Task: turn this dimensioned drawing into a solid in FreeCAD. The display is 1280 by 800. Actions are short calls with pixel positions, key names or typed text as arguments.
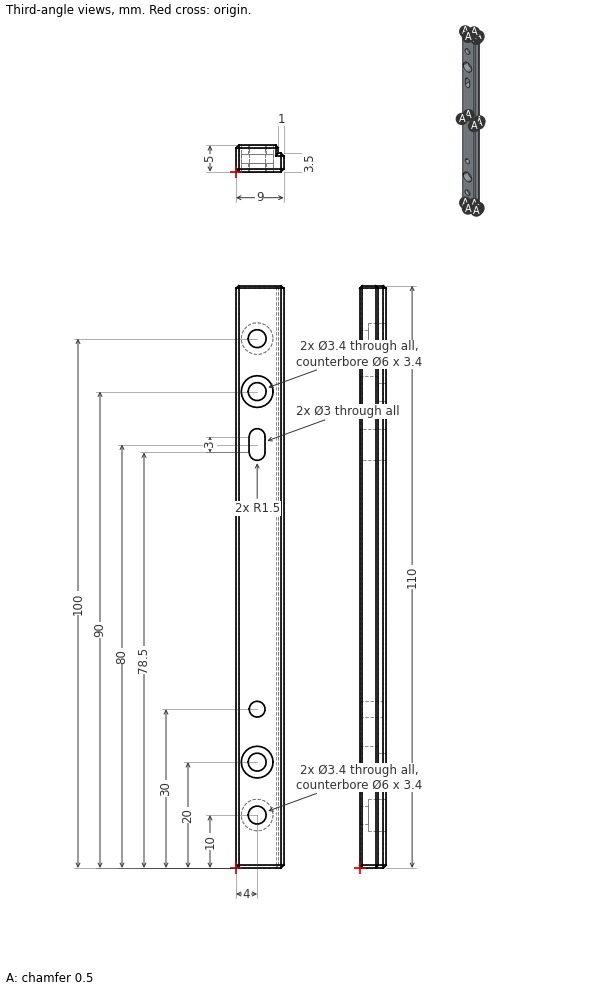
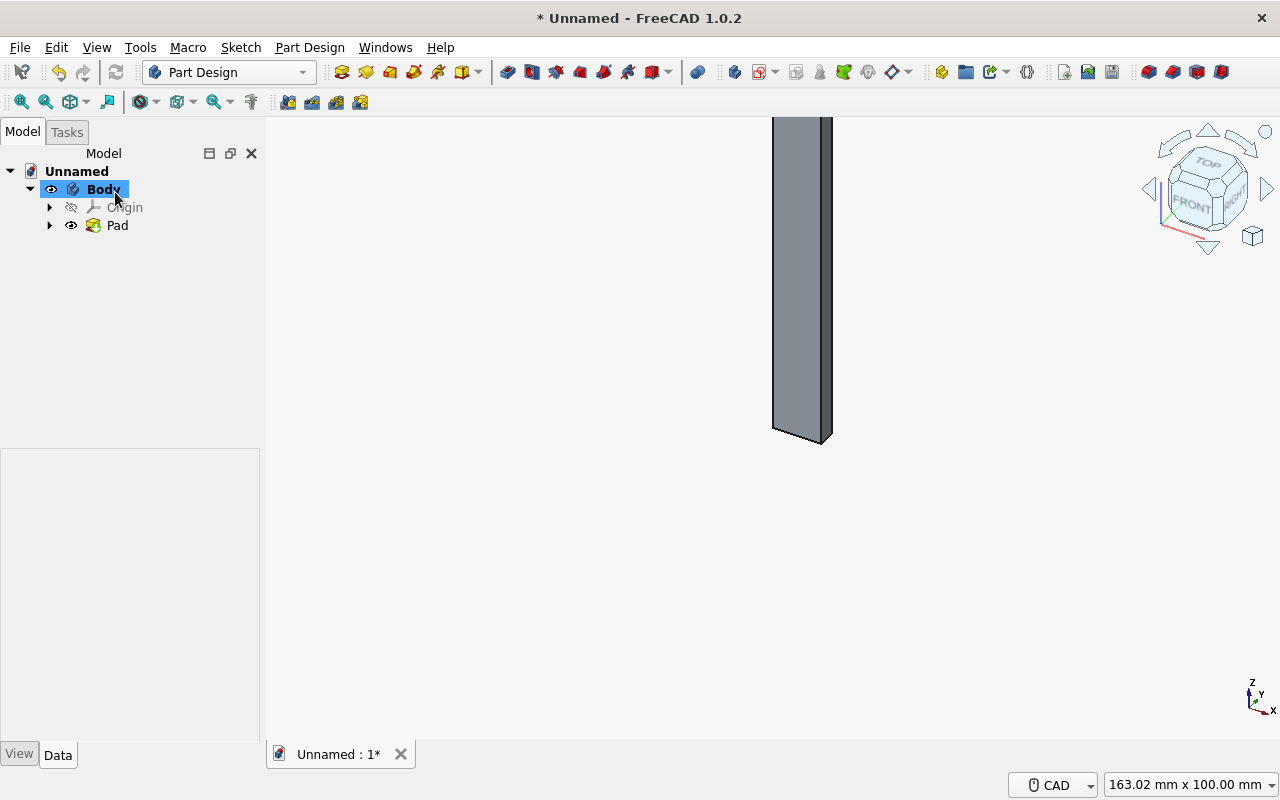
key(v)
key(f)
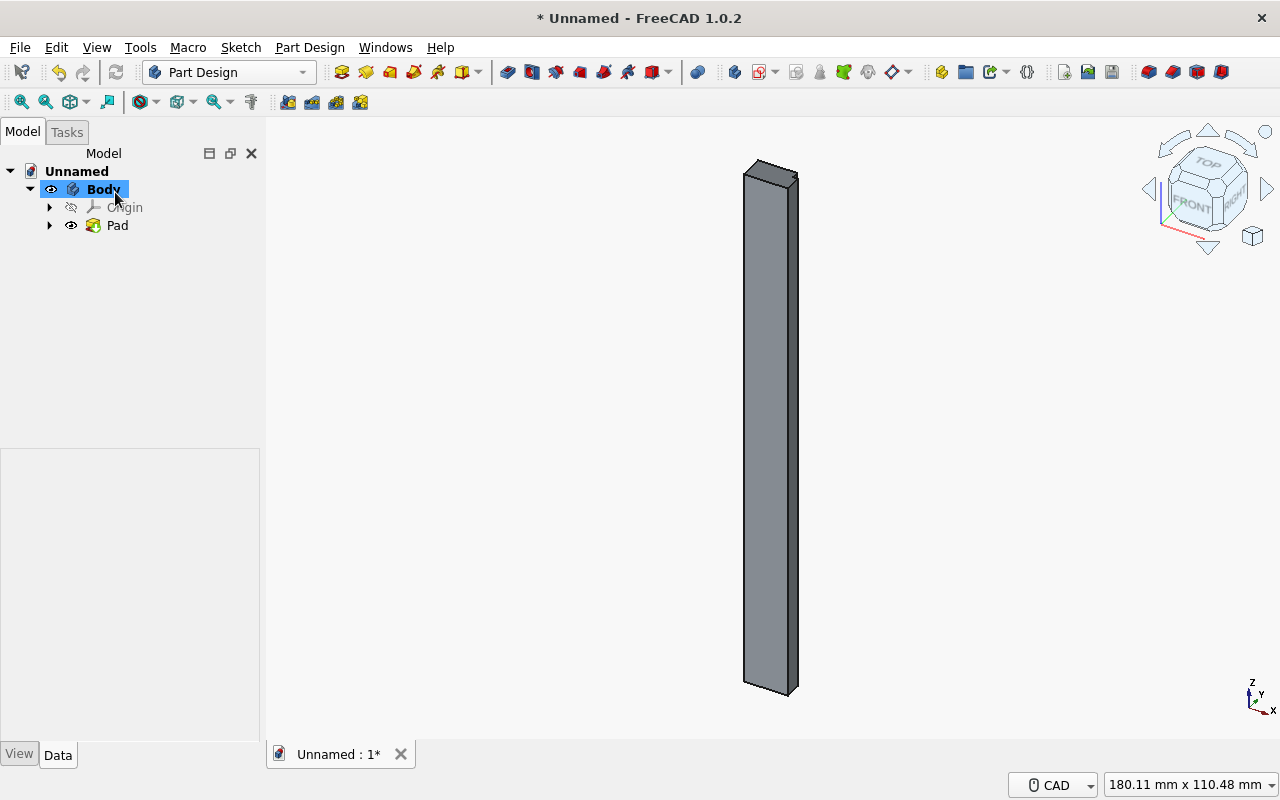
key(4)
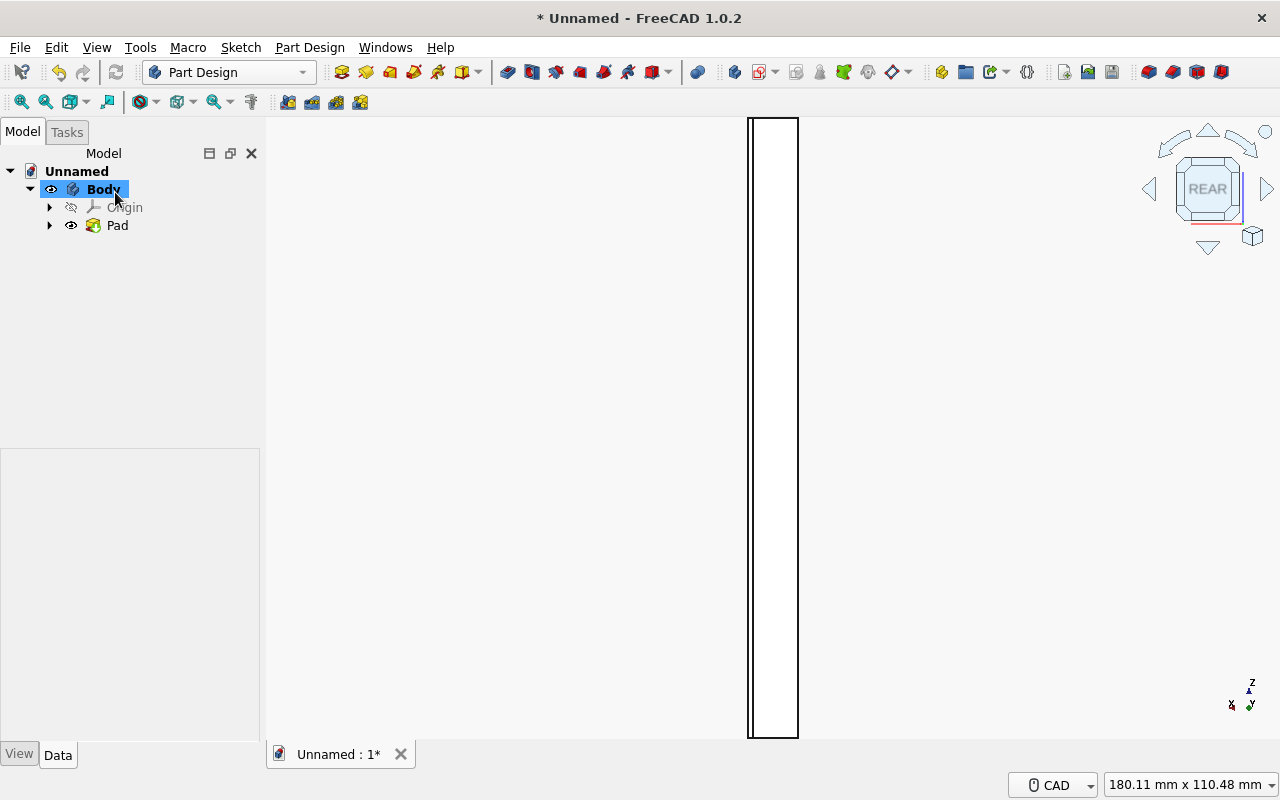
click(776, 162)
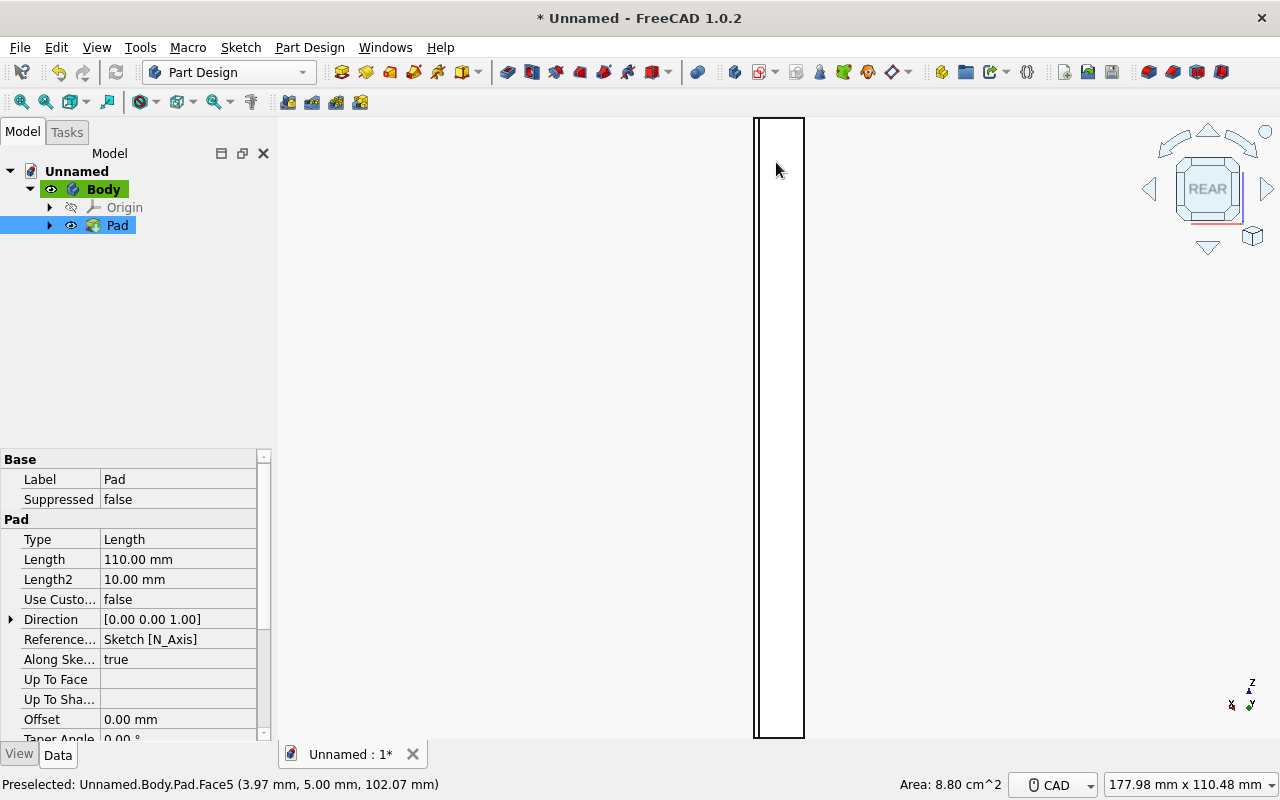
click(760, 72)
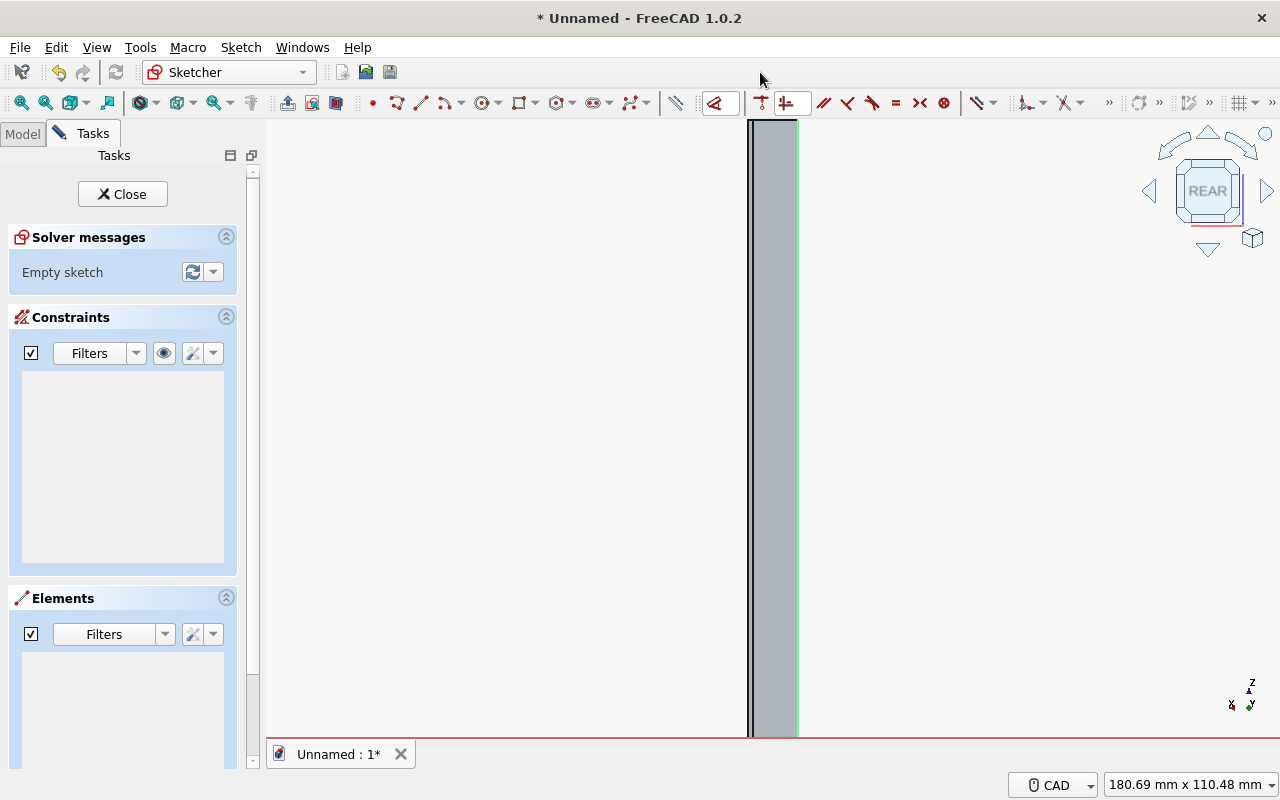
scroll(546, 382, down, 2)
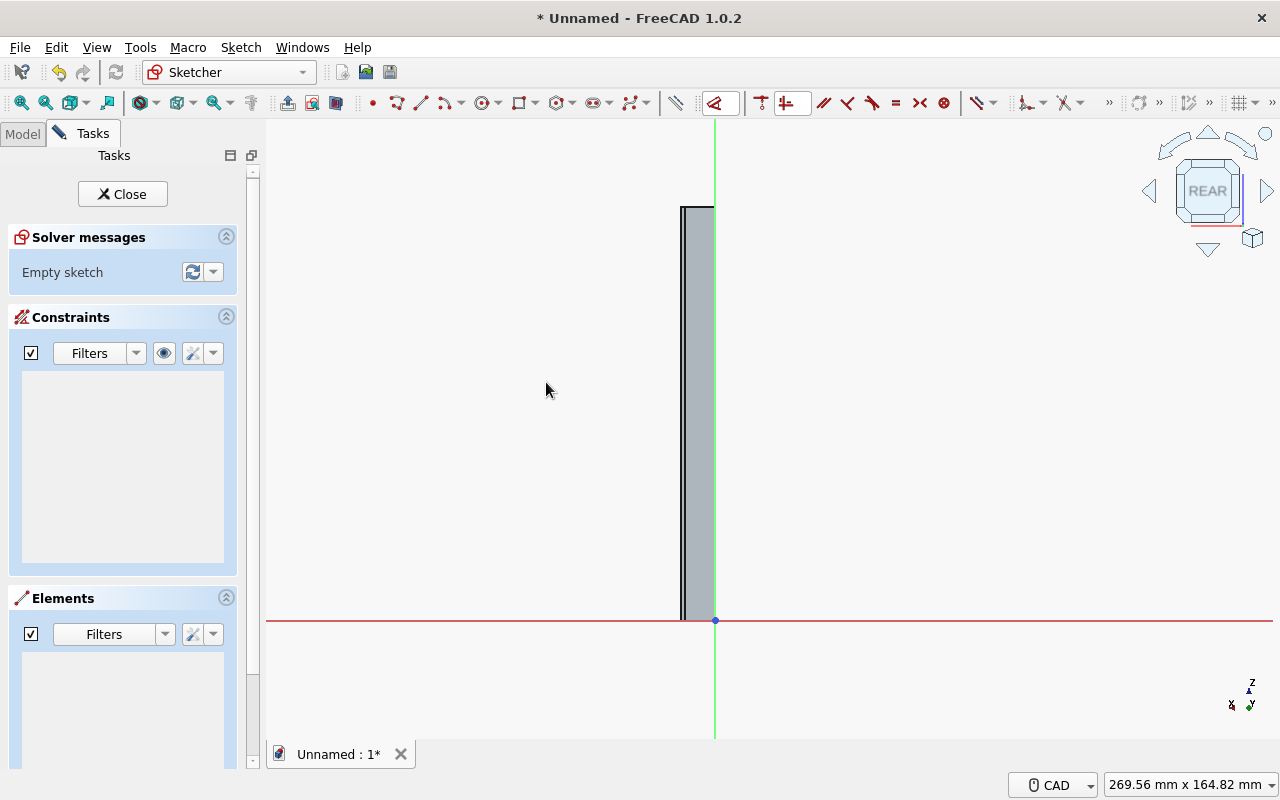
key(g)
key(c)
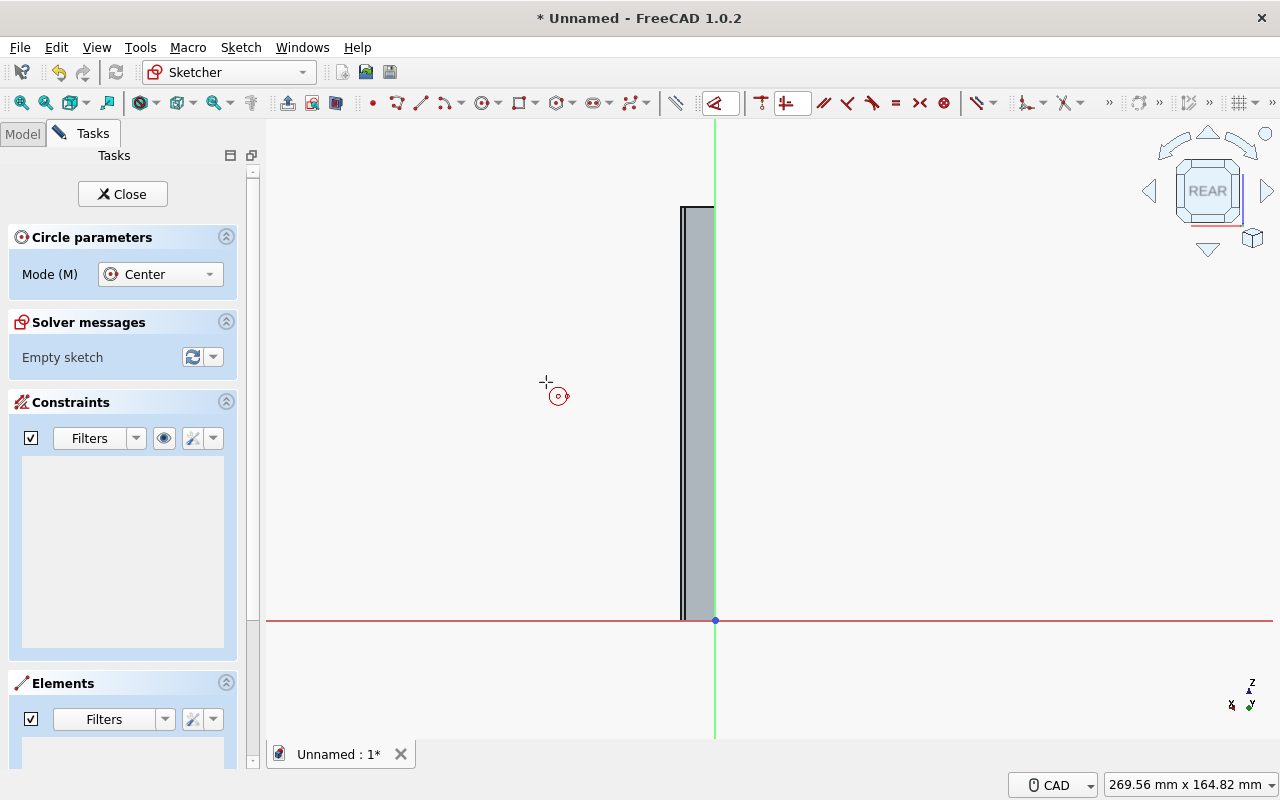
scroll(700, 583, up, 7)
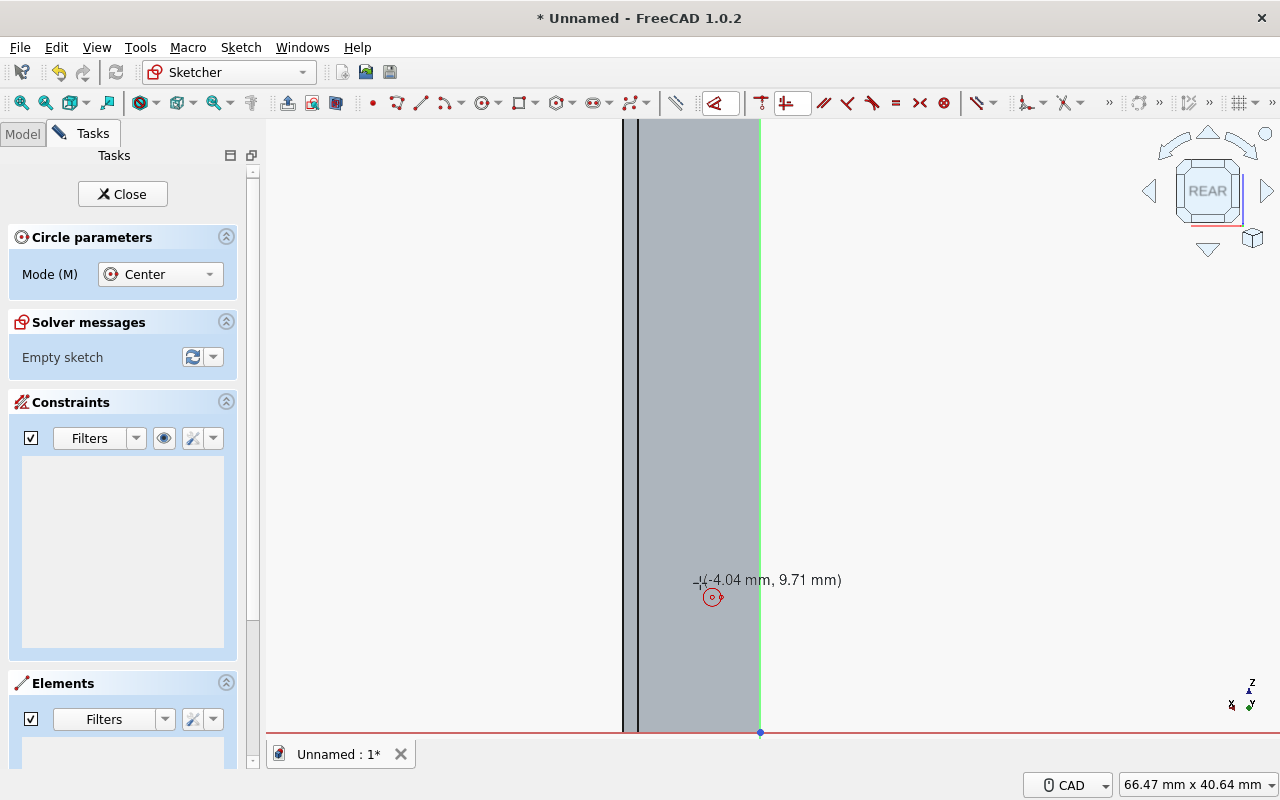
scroll(700, 583, down, 7)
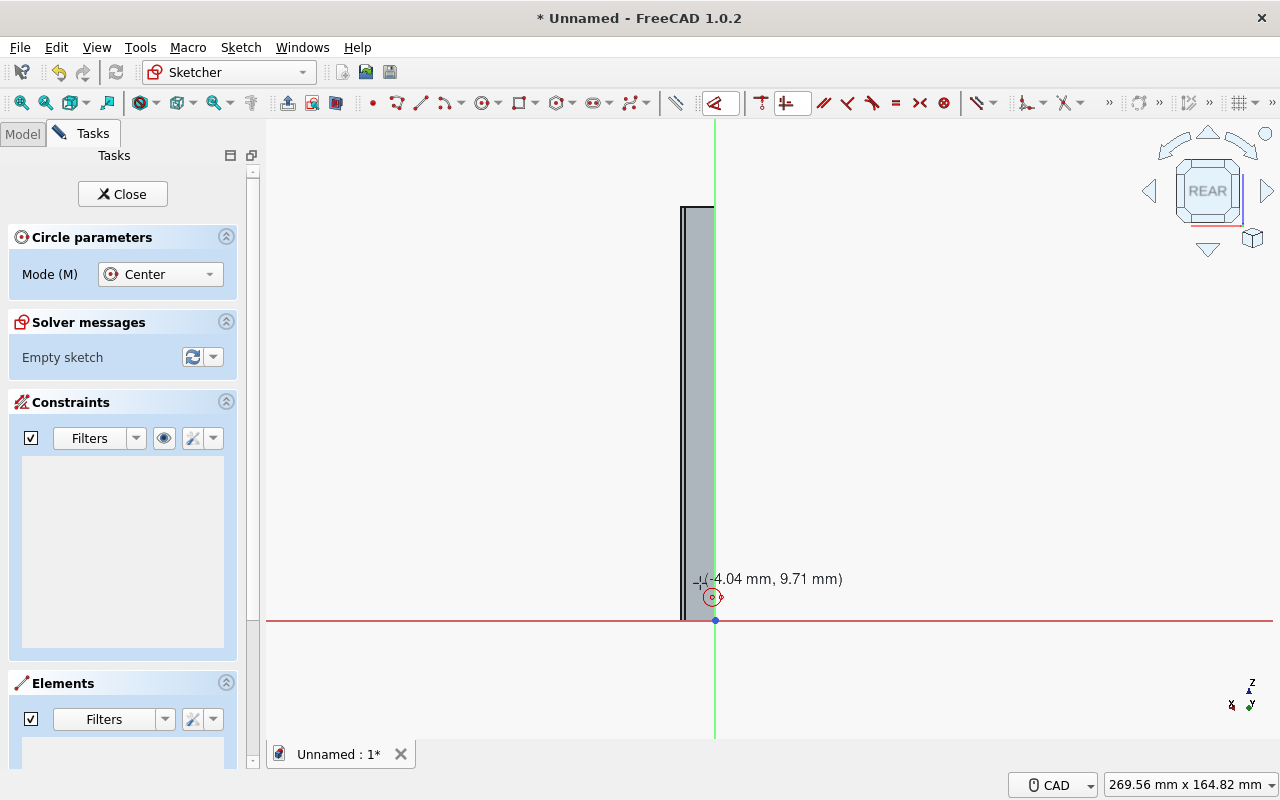
click(700, 583)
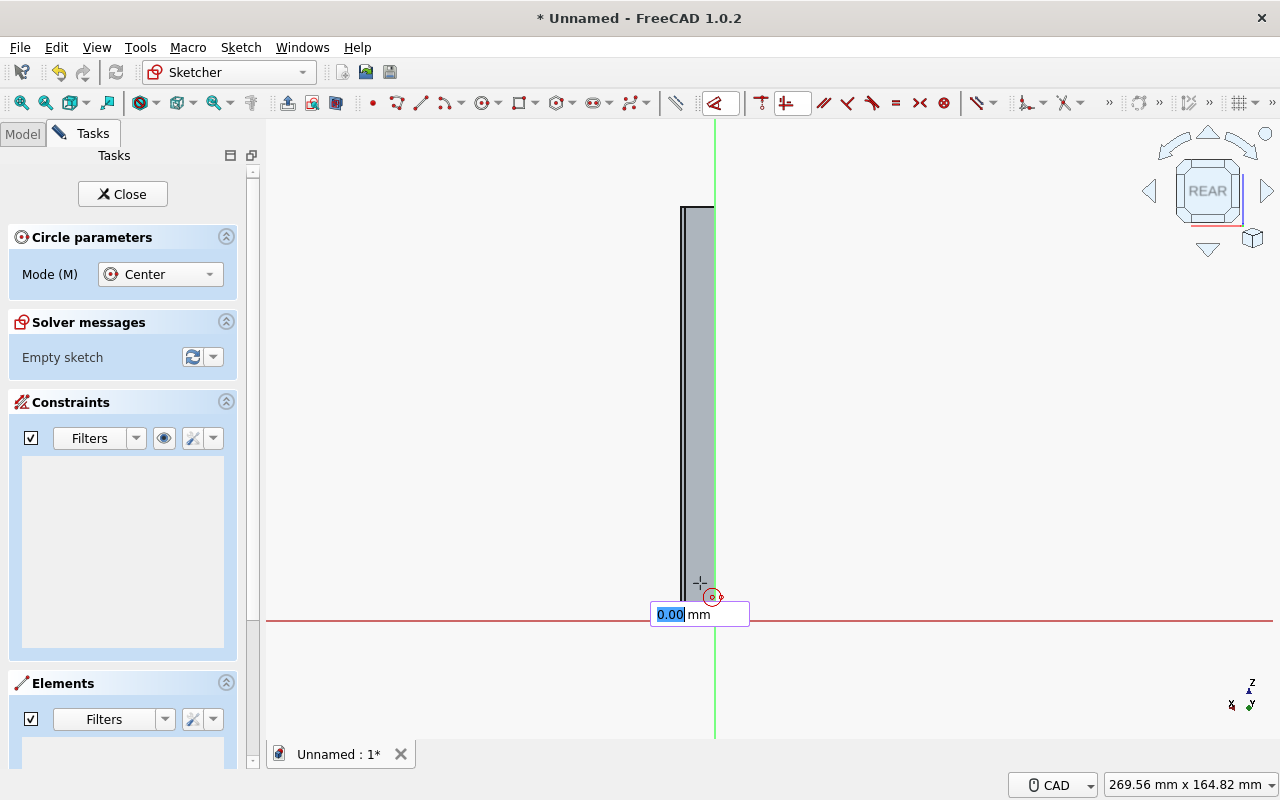
scroll(696, 578, up, 5)